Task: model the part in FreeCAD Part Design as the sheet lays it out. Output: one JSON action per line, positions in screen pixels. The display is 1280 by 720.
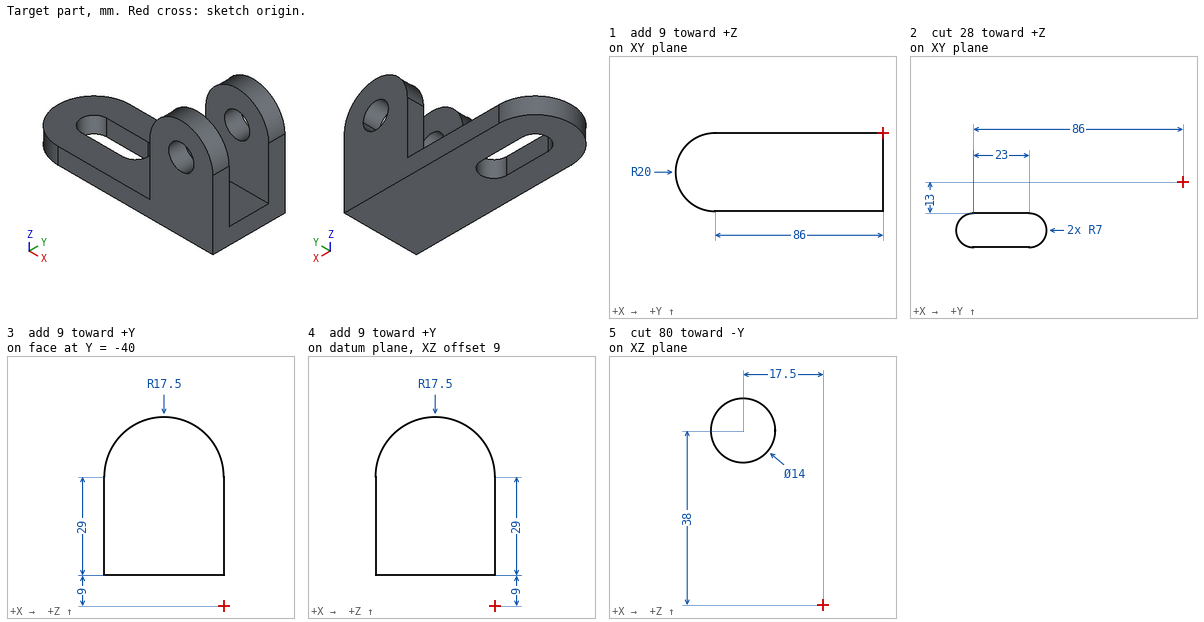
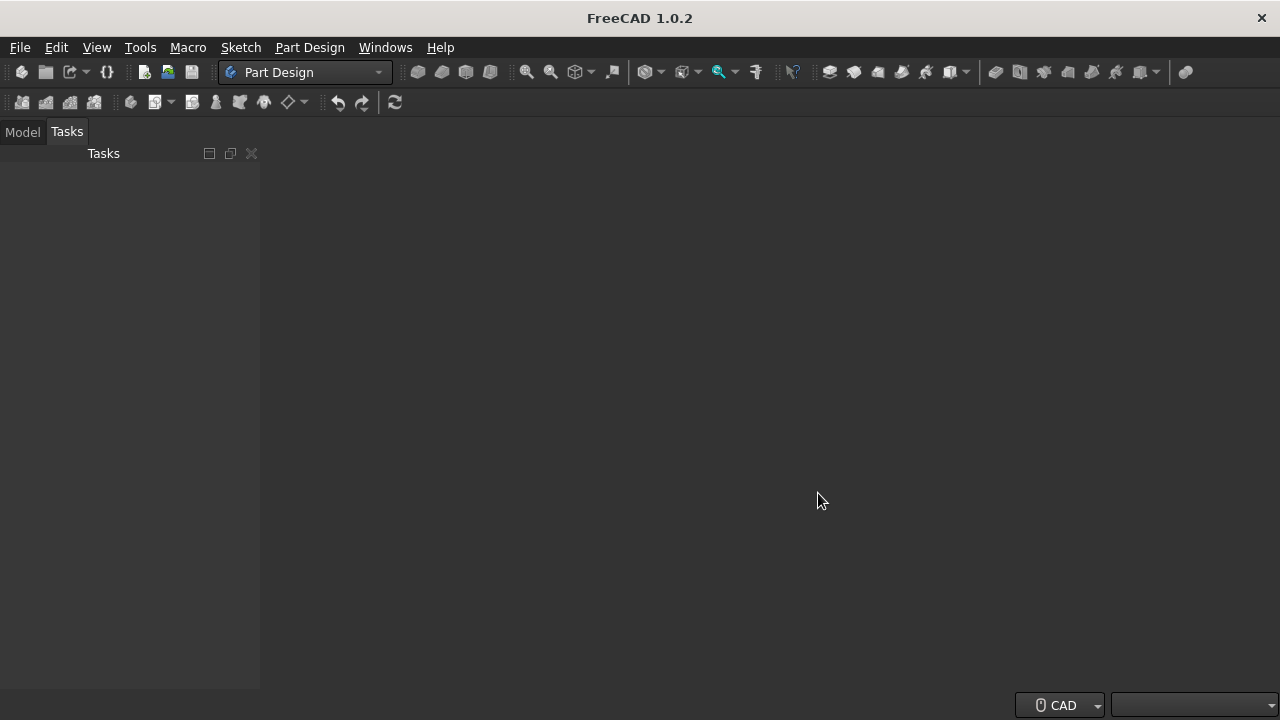
{"action": "left_click", "coordinate": [144, 72]}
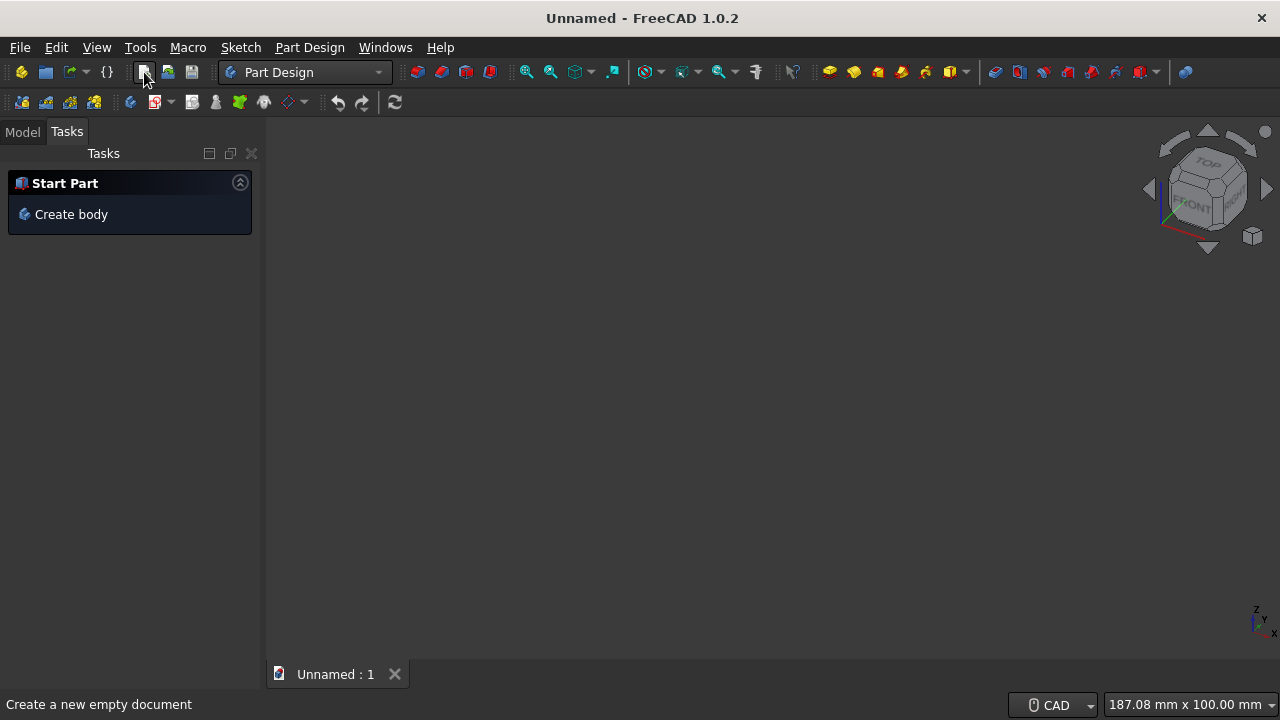
{"action": "left_click", "coordinate": [156, 102]}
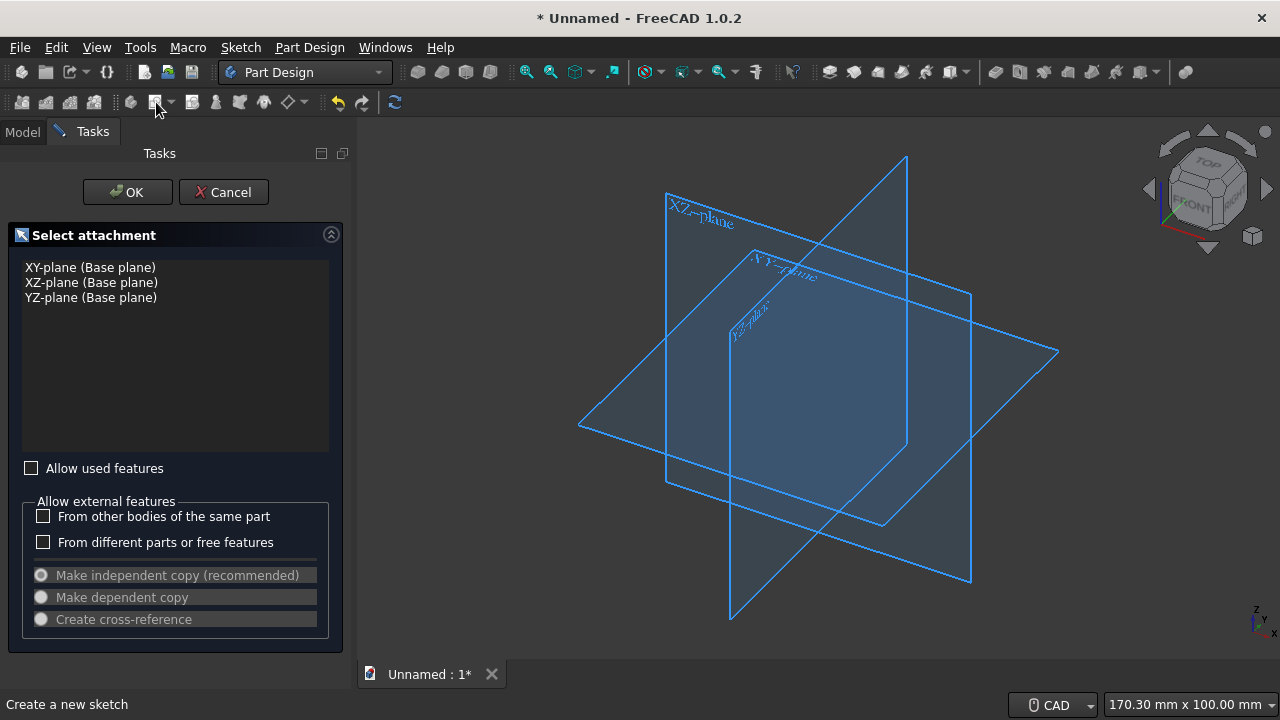
{"action": "left_click", "coordinate": [82, 268]}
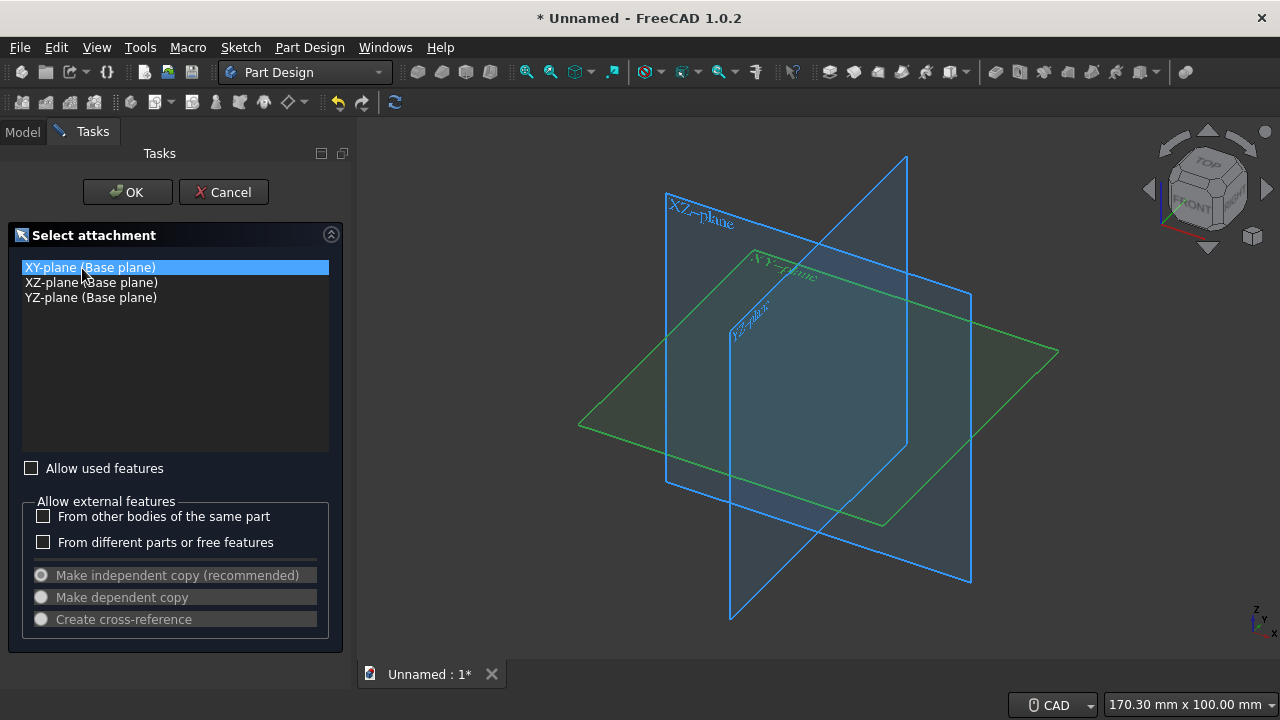
{"action": "left_click", "coordinate": [128, 192]}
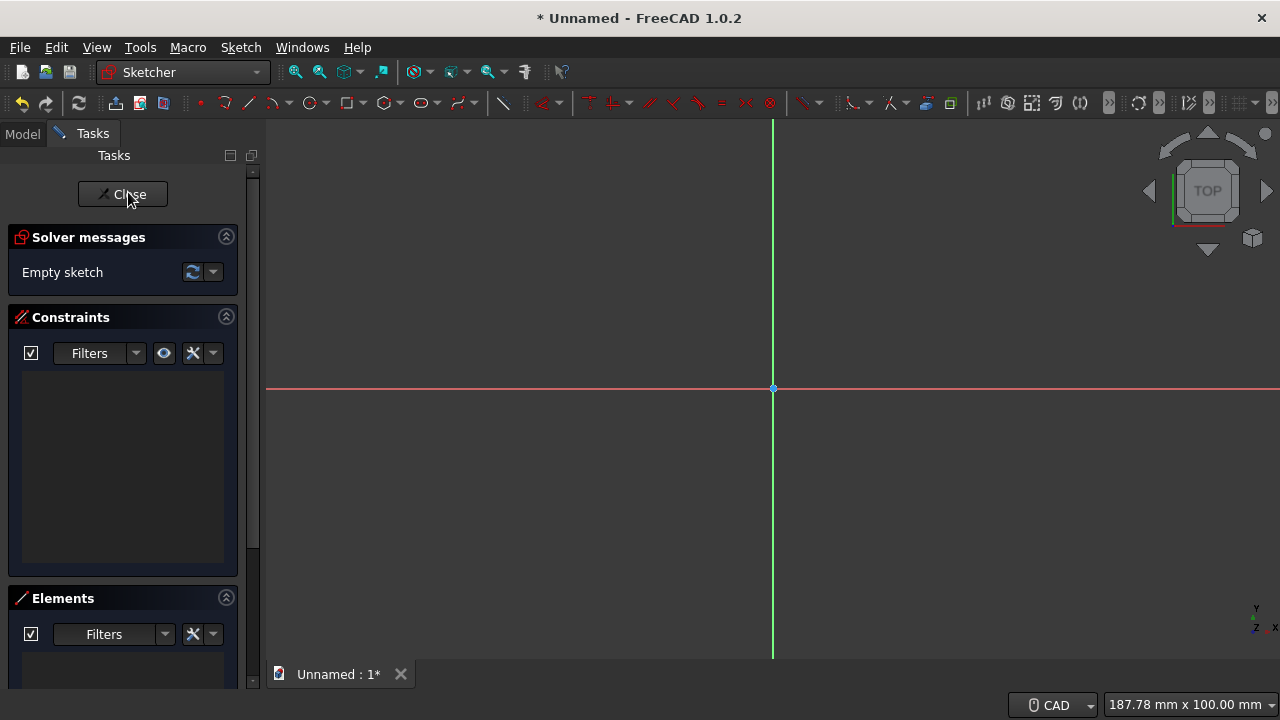
{"action": "scroll", "coordinate": [1115, 147], "scroll_direction": "down", "scroll_amount": 1}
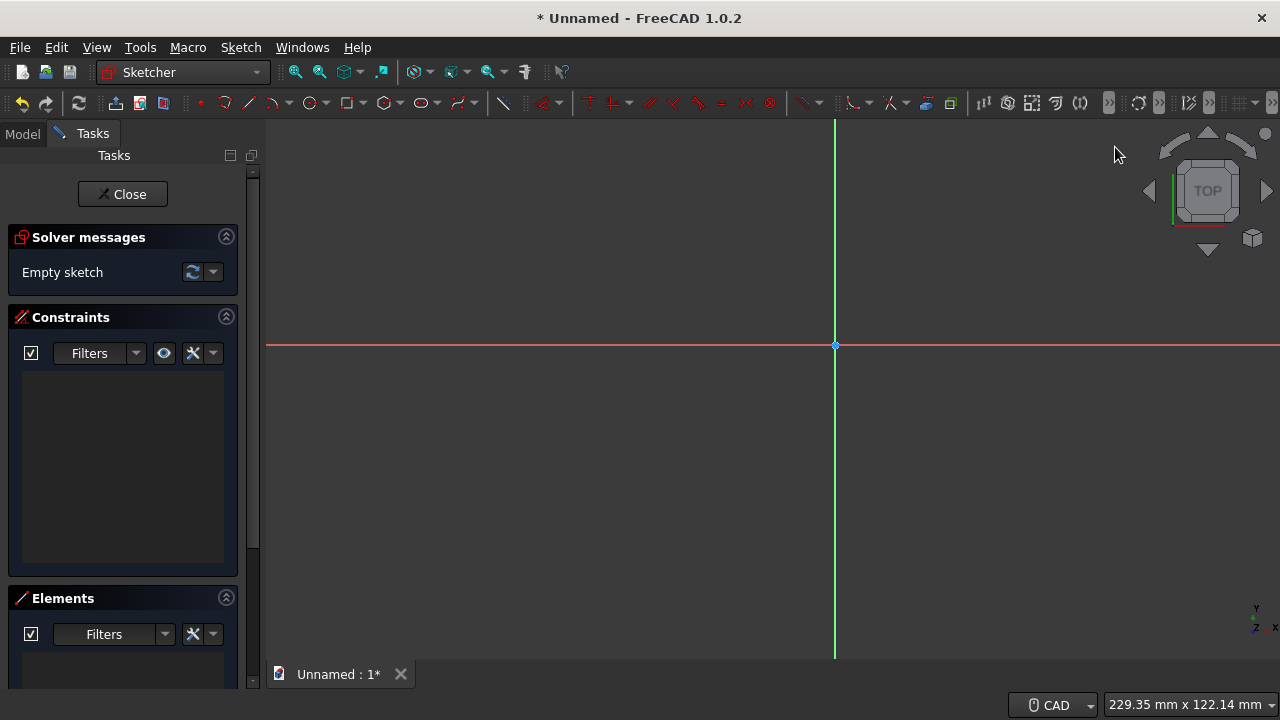
{"action": "left_click", "coordinate": [226, 104]}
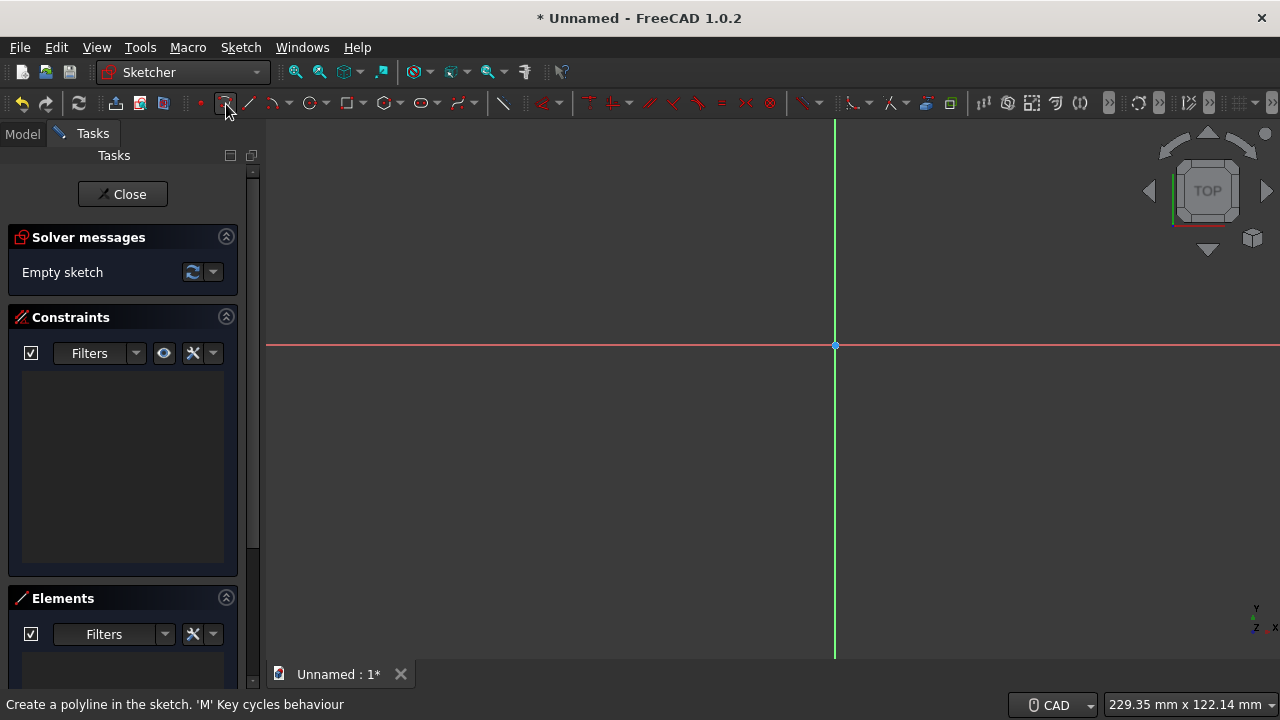
{"action": "left_click", "coordinate": [455, 522]}
{"action": "left_click", "coordinate": [835, 522]}
{"action": "left_click", "coordinate": [835, 345]}
{"action": "left_click", "coordinate": [455, 354]}
{"action": "right_click", "coordinate": [455, 354]}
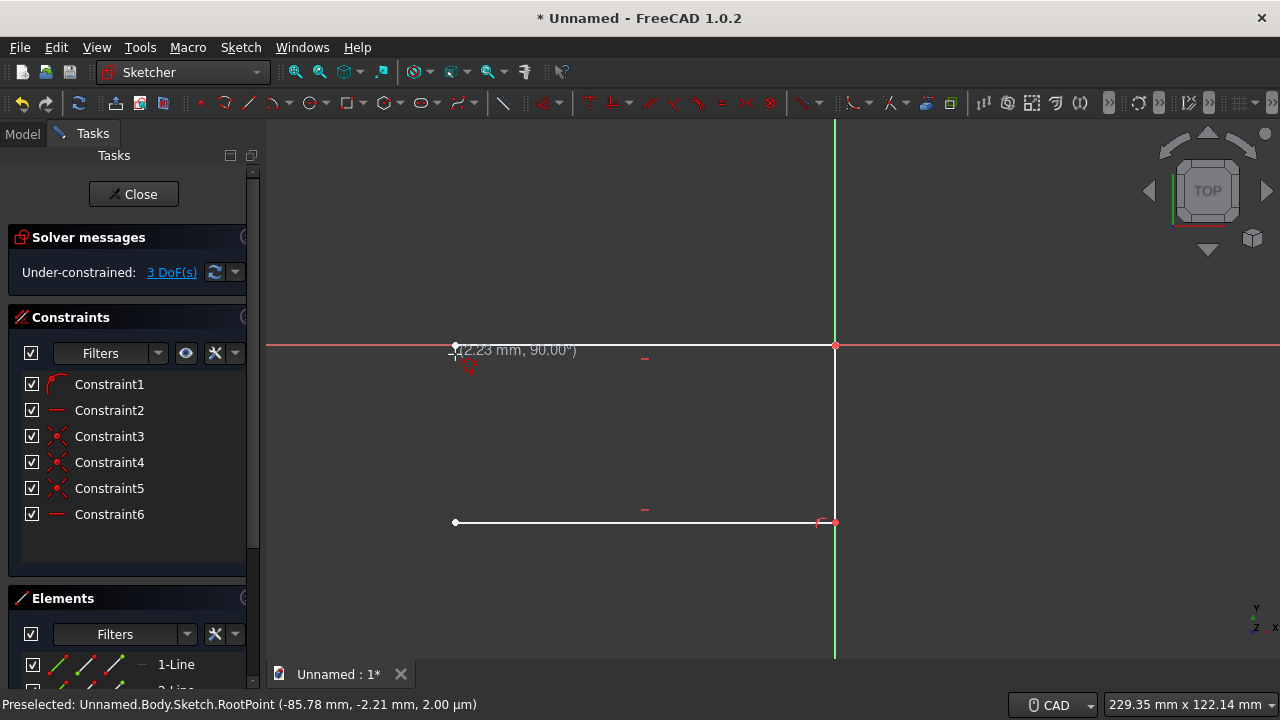
{"action": "key", "text": "g 3 a"}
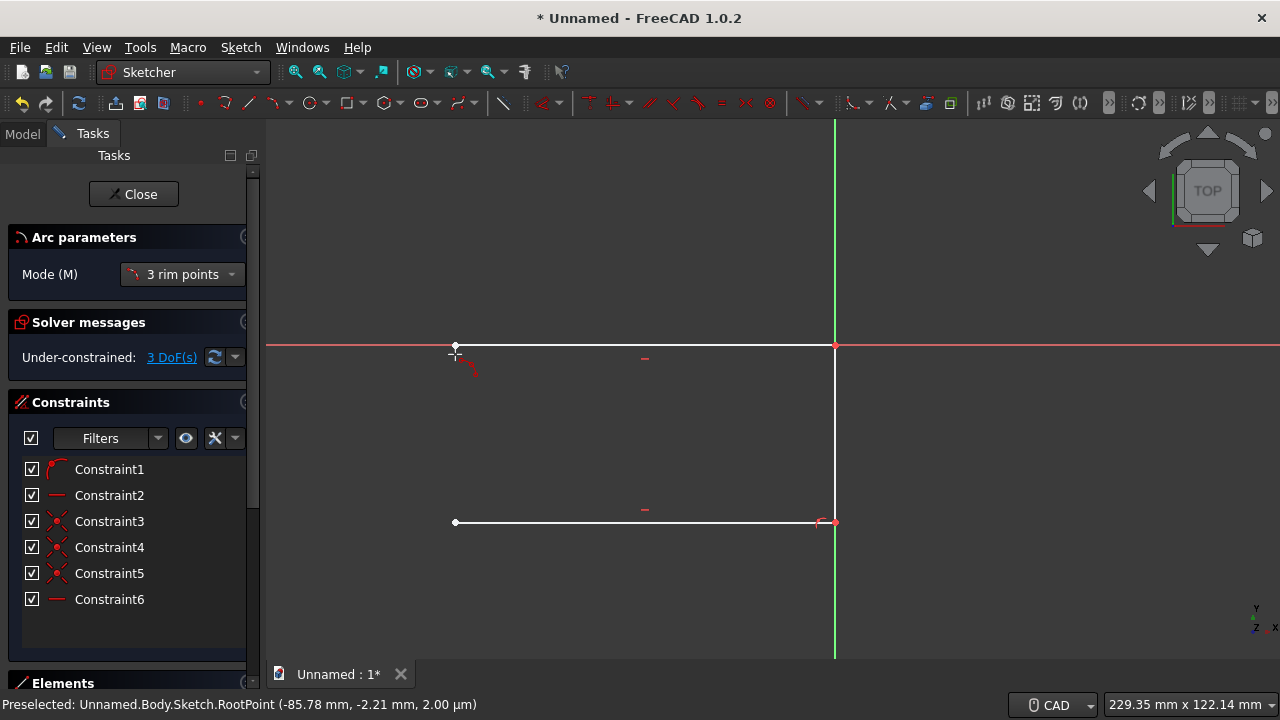
{"action": "left_click", "coordinate": [455, 345]}
{"action": "left_click", "coordinate": [455, 523]}
{"action": "left_click", "coordinate": [367, 434]}
{"action": "key", "text": "Escape"}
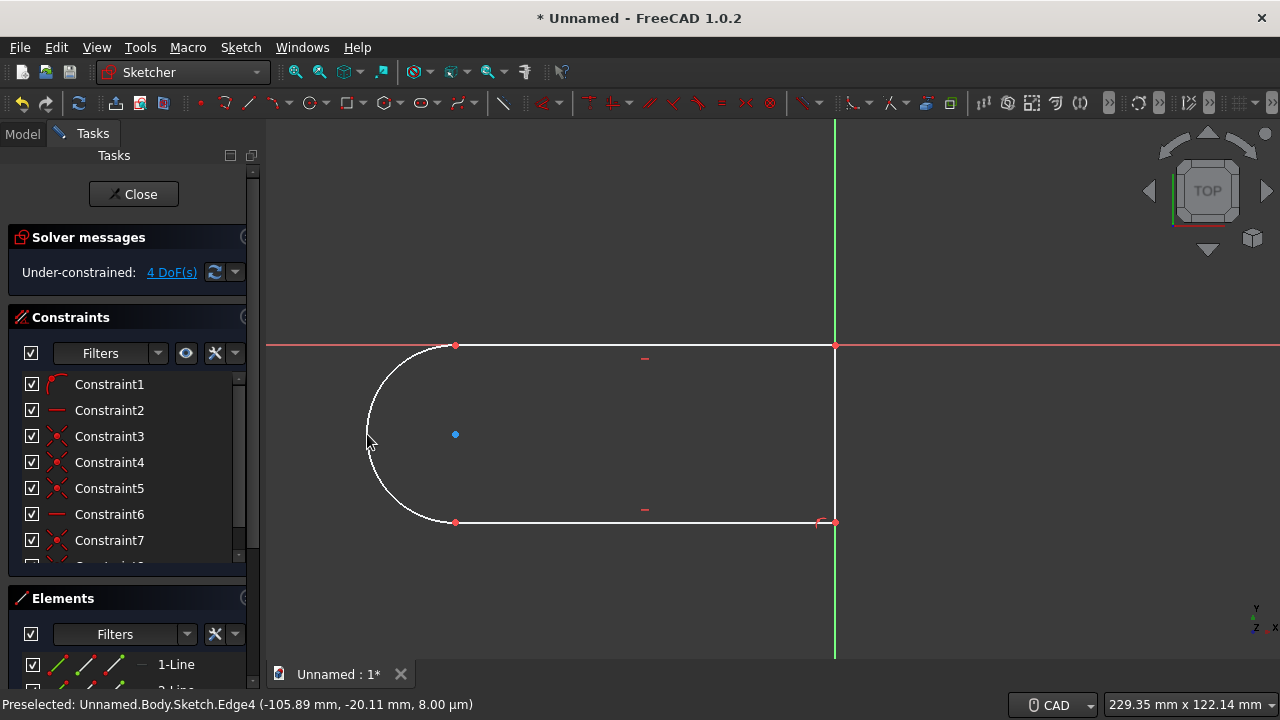
{"action": "left_click", "coordinate": [569, 523]}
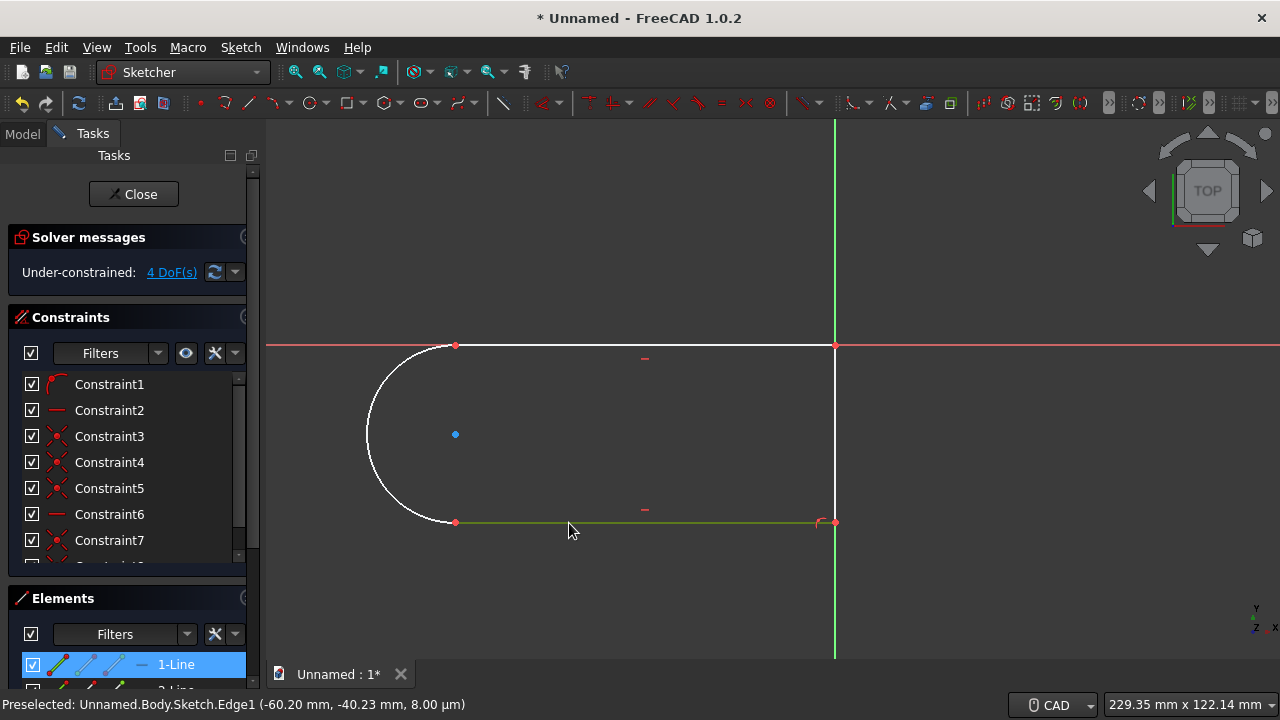
{"action": "left_click", "coordinate": [384, 382]}